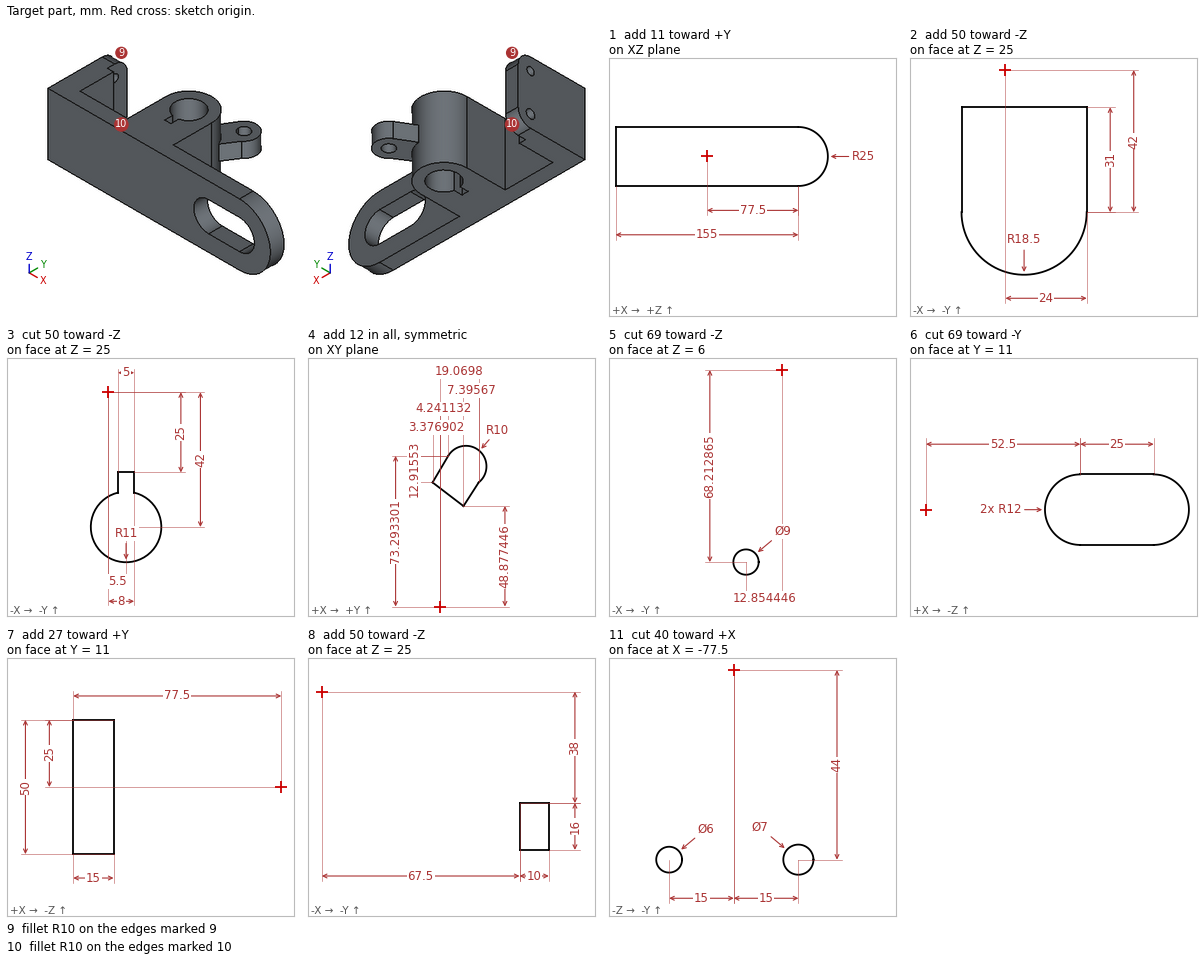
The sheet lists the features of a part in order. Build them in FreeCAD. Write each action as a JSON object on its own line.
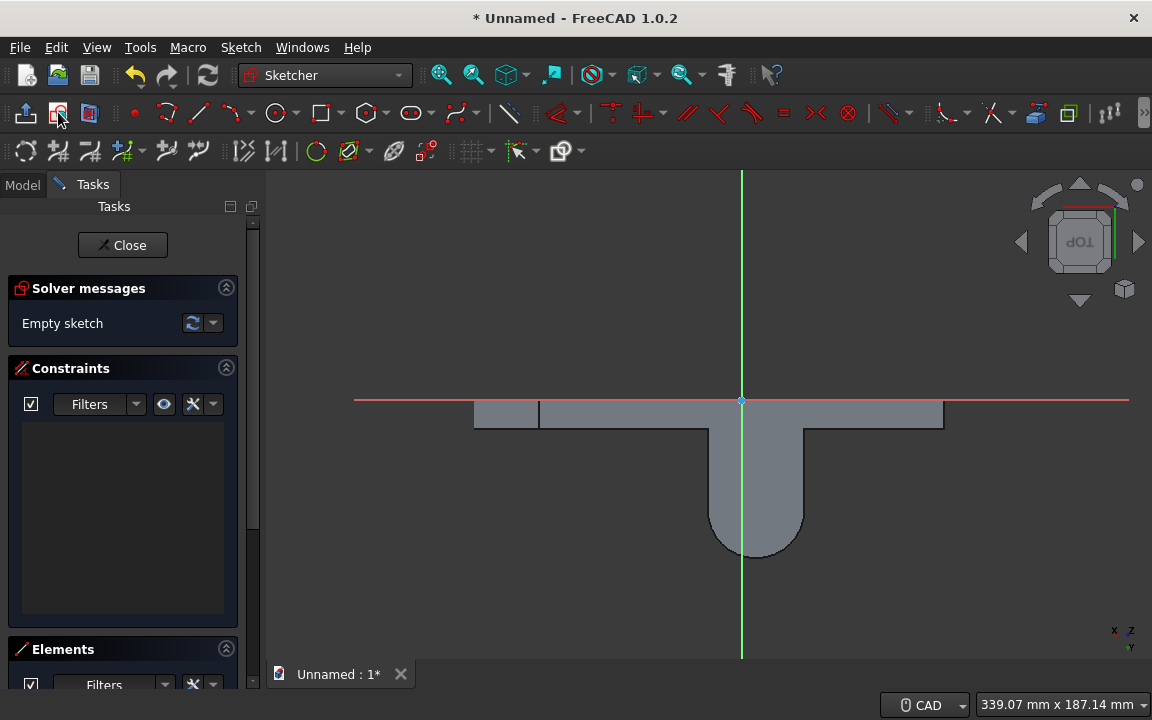
{"action": "scroll", "coordinate": [843, 514], "scroll_direction": "up", "scroll_amount": 4}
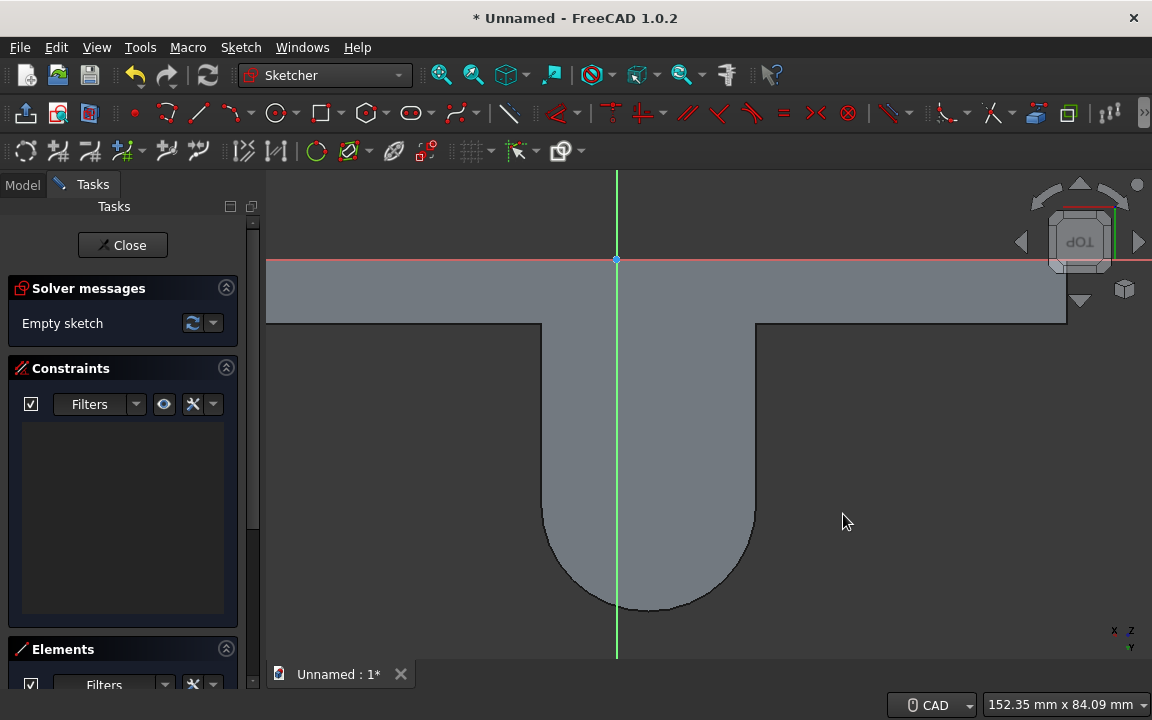
{"action": "left_click", "coordinate": [168, 114]}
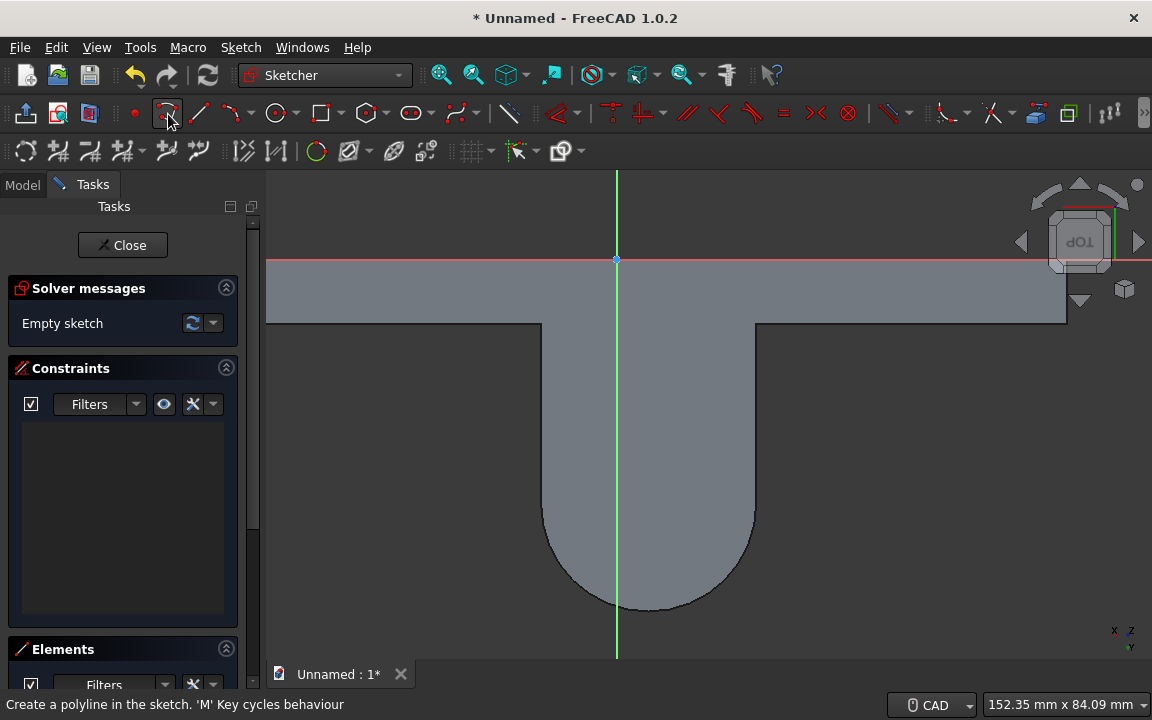
{"action": "left_click", "coordinate": [663, 442]}
{"action": "left_click", "coordinate": [663, 405]}
{"action": "left_click", "coordinate": [634, 405]}
{"action": "left_click", "coordinate": [634, 442]}
{"action": "right_click", "coordinate": [634, 442]}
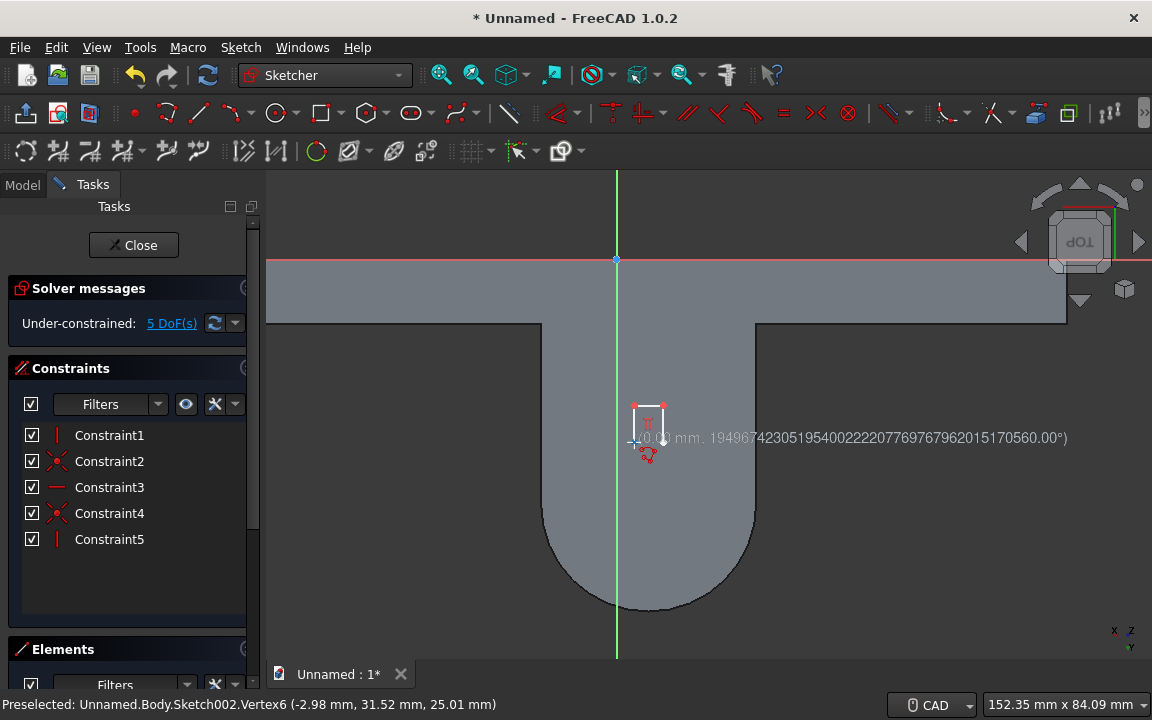
{"action": "left_click", "coordinate": [232, 114]}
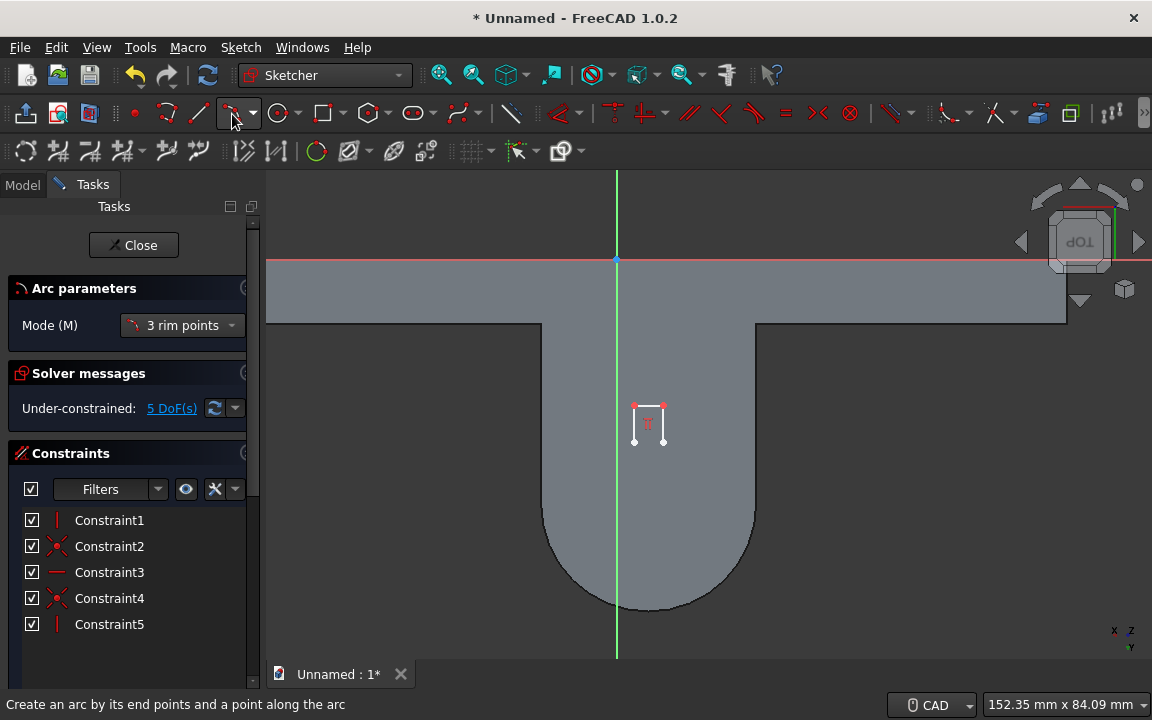
{"action": "left_click", "coordinate": [634, 443]}
{"action": "left_click", "coordinate": [663, 443]}
{"action": "left_click", "coordinate": [649, 568]}
{"action": "key", "text": "Escape"}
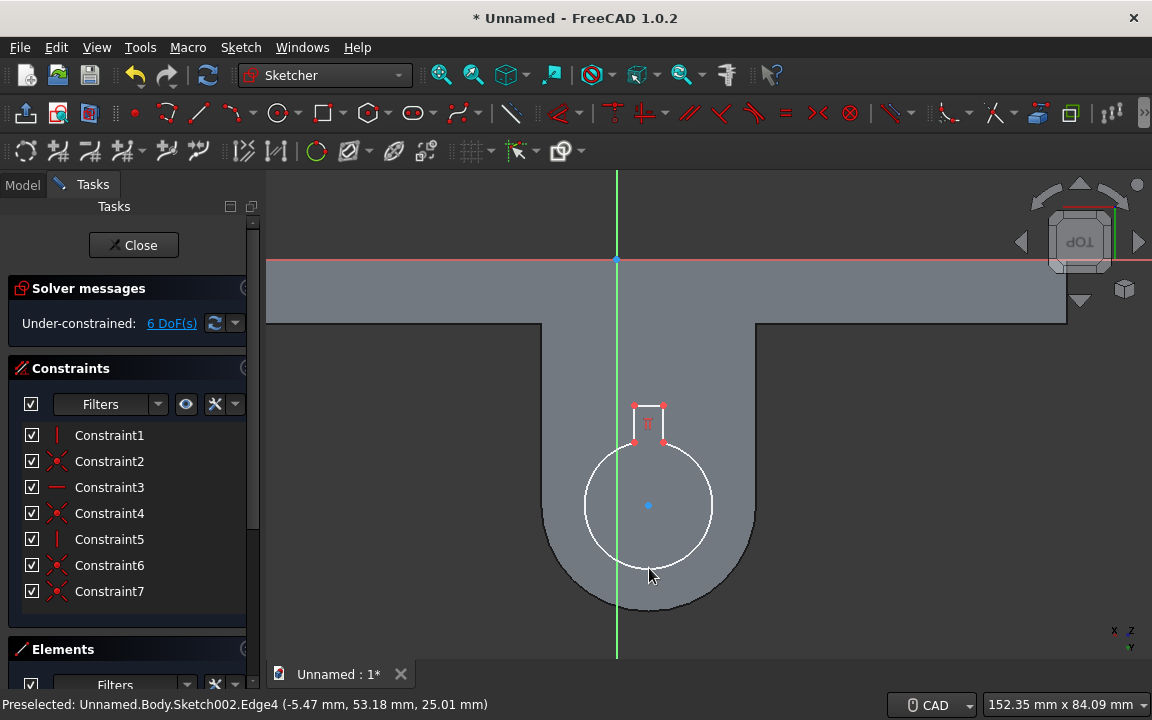
{"action": "left_click", "coordinate": [558, 114]}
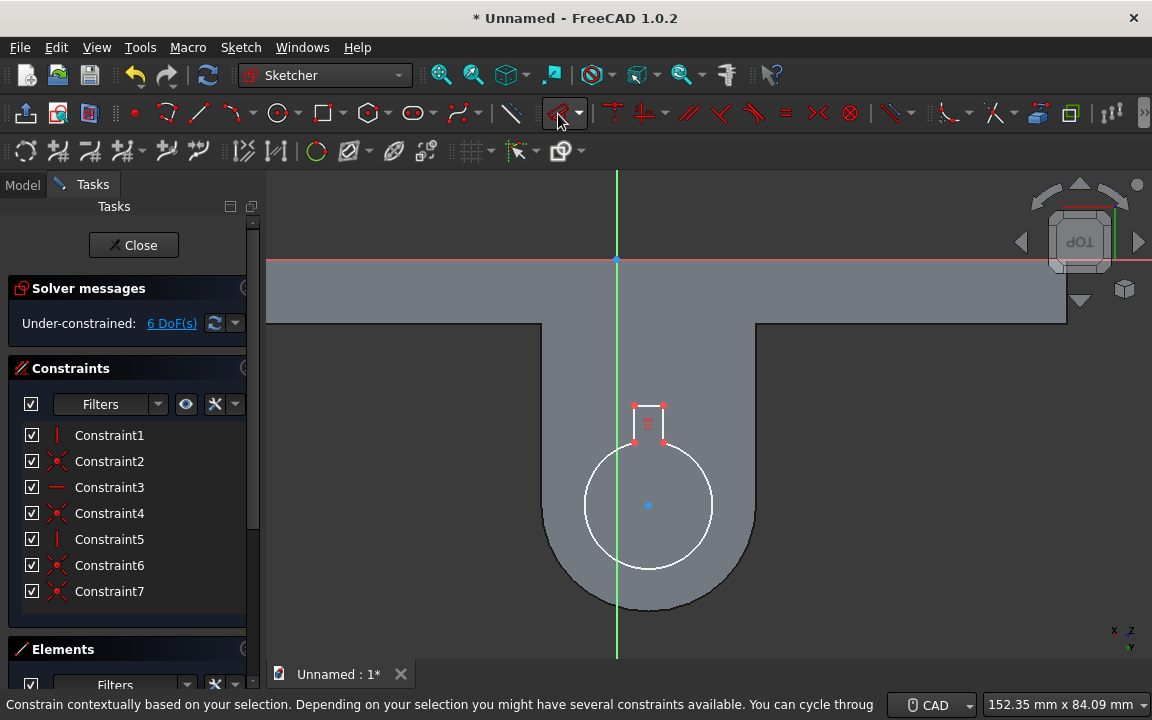
{"action": "left_click", "coordinate": [590, 530]}
{"action": "left_click", "coordinate": [561, 543]}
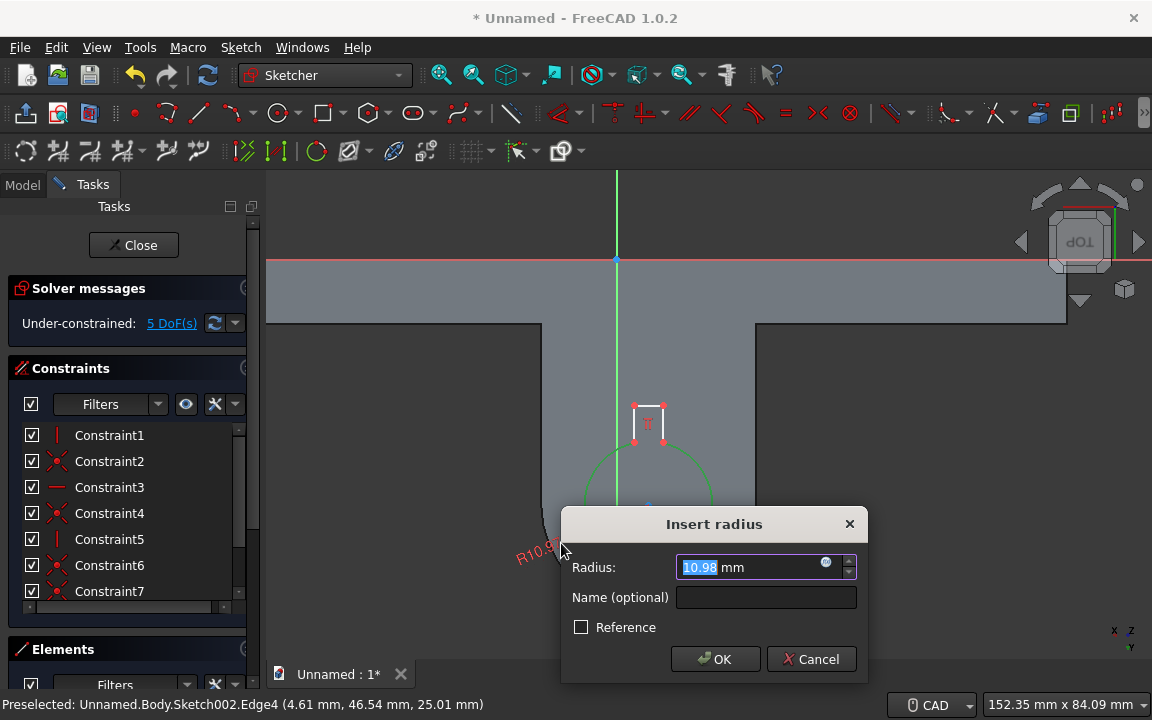
{"action": "type", "text": "11"}
{"action": "key", "text": "Return"}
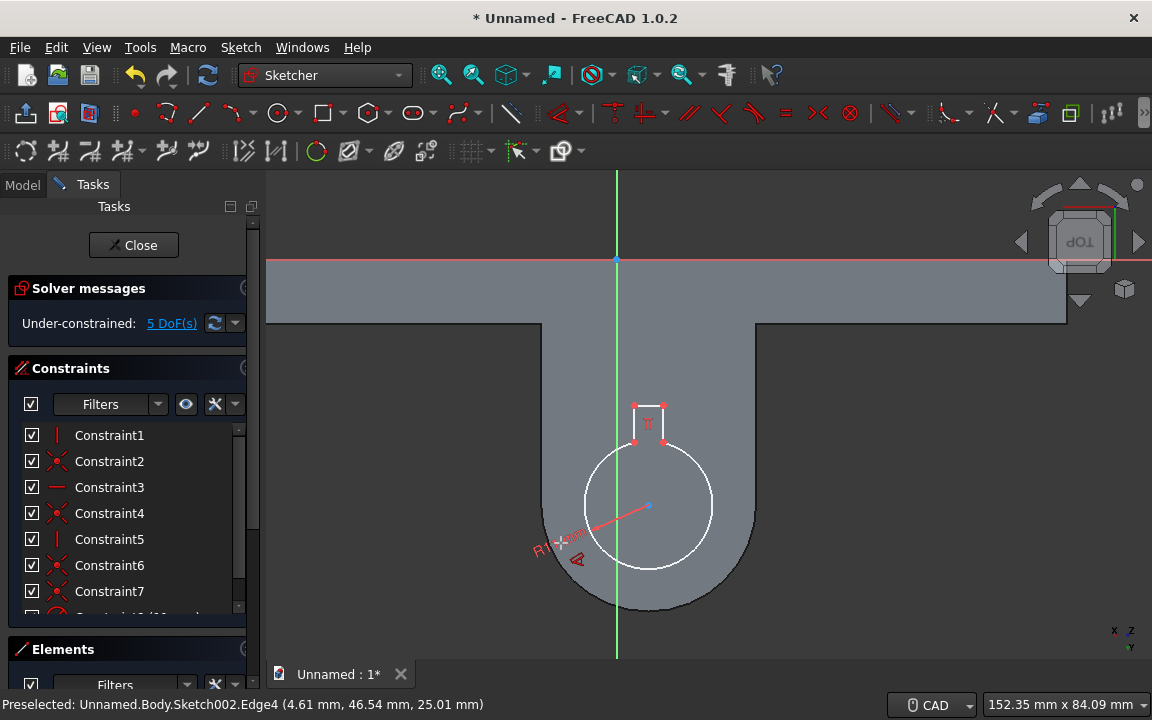
{"action": "scroll", "coordinate": [651, 406], "scroll_direction": "up", "scroll_amount": 2}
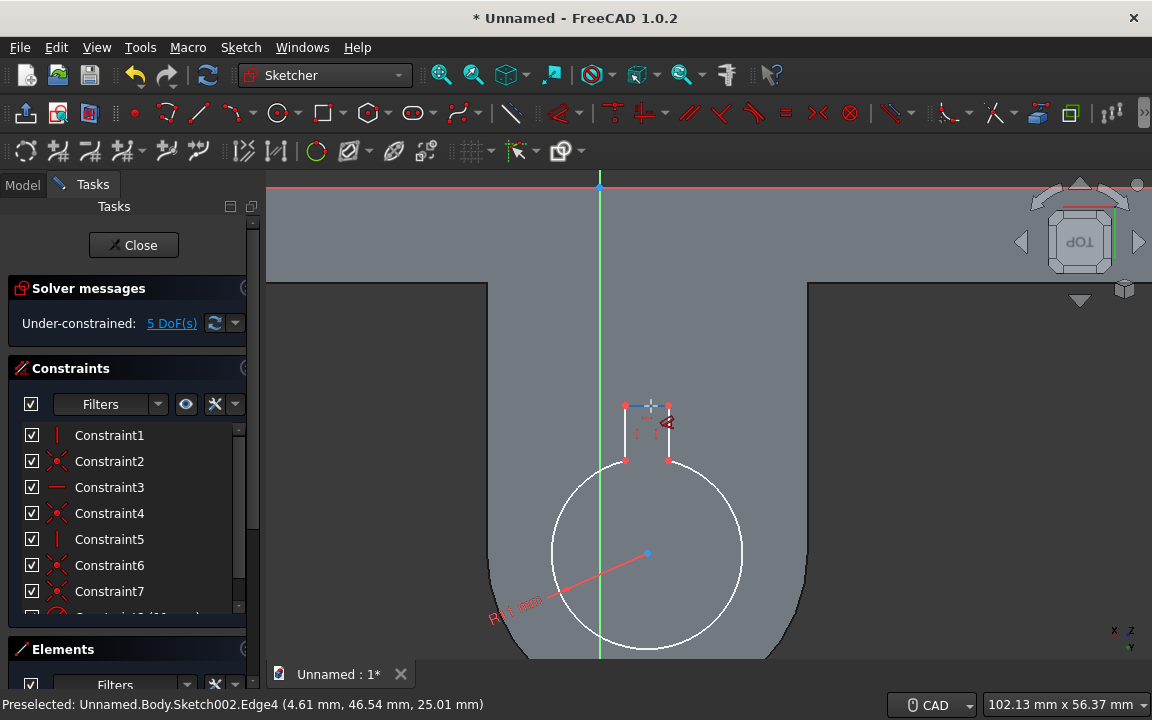
{"action": "left_click", "coordinate": [651, 406]}
{"action": "left_click", "coordinate": [647, 372]}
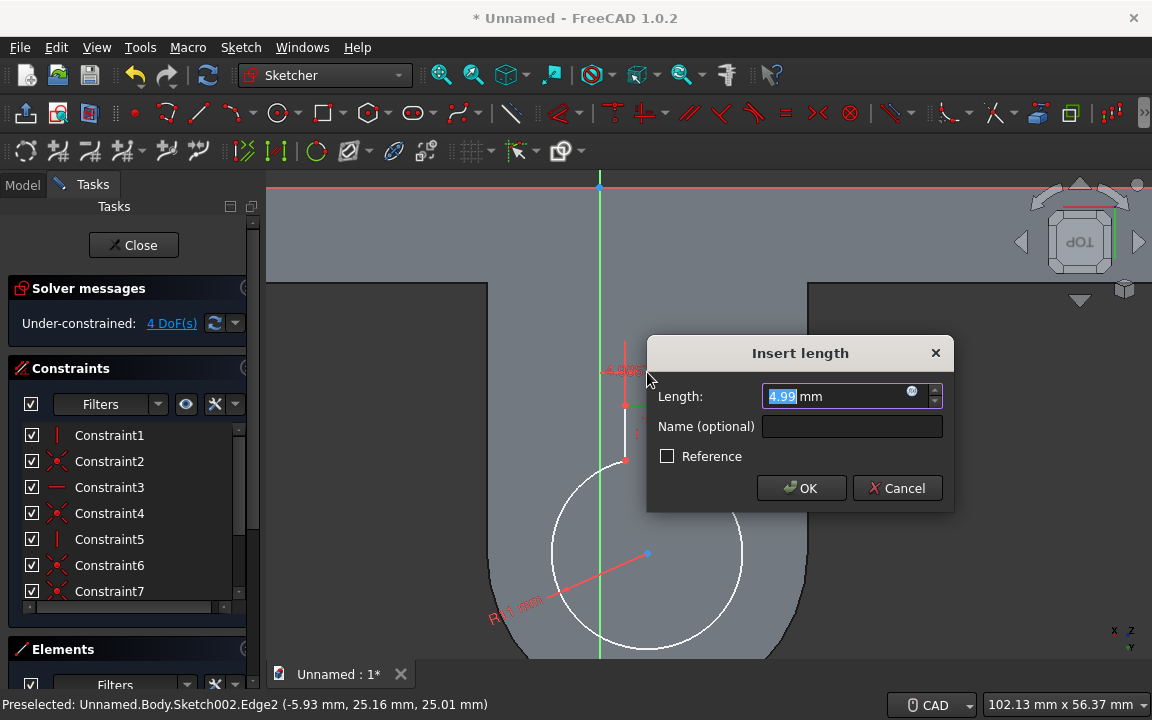
{"action": "type", "text": "5"}
{"action": "key", "text": "Return"}